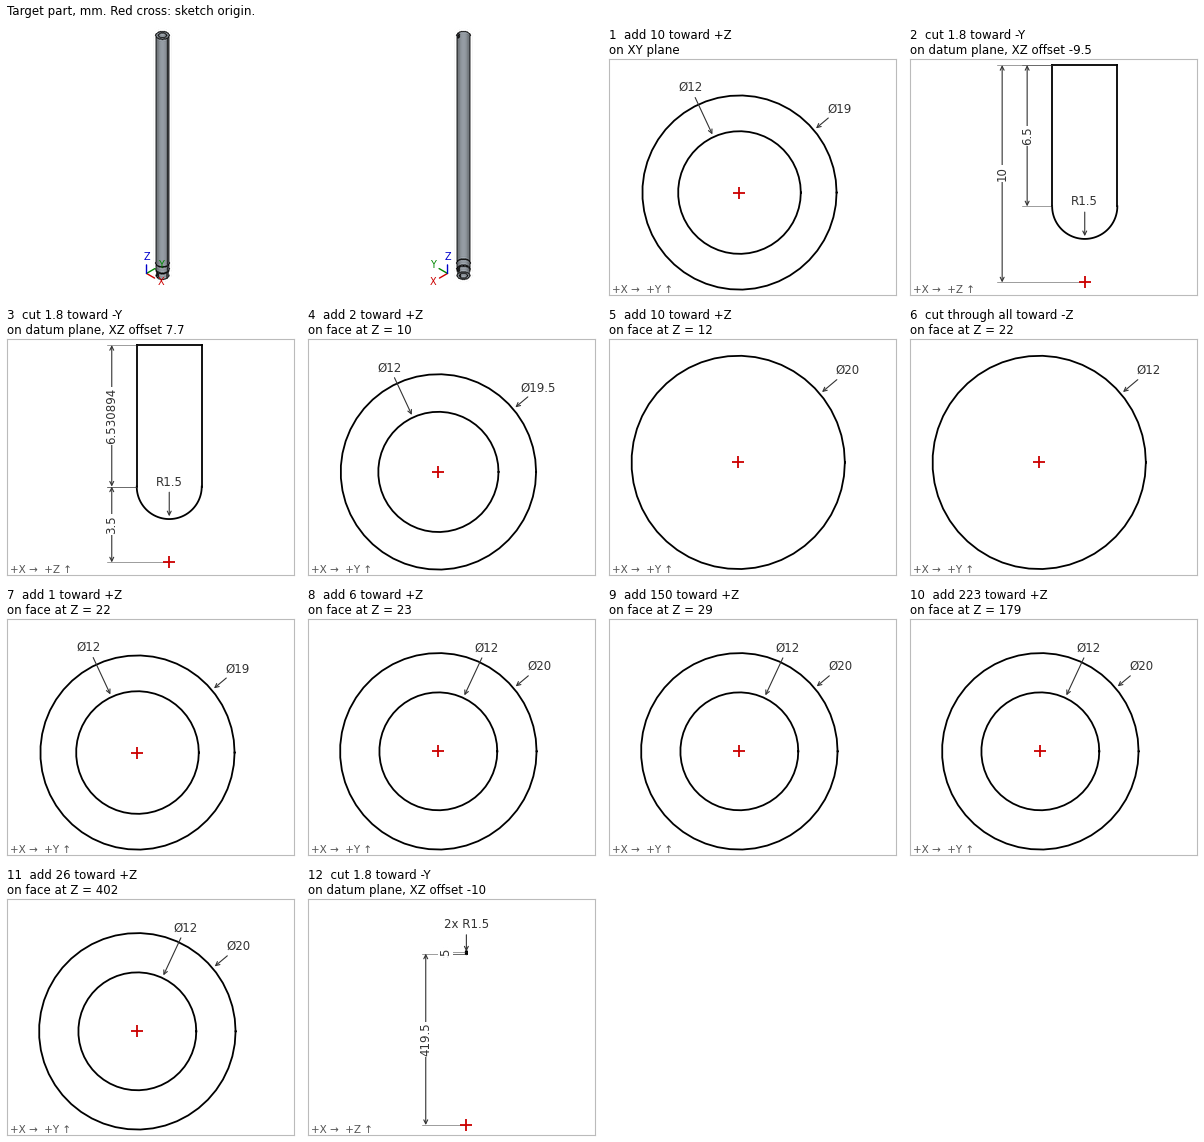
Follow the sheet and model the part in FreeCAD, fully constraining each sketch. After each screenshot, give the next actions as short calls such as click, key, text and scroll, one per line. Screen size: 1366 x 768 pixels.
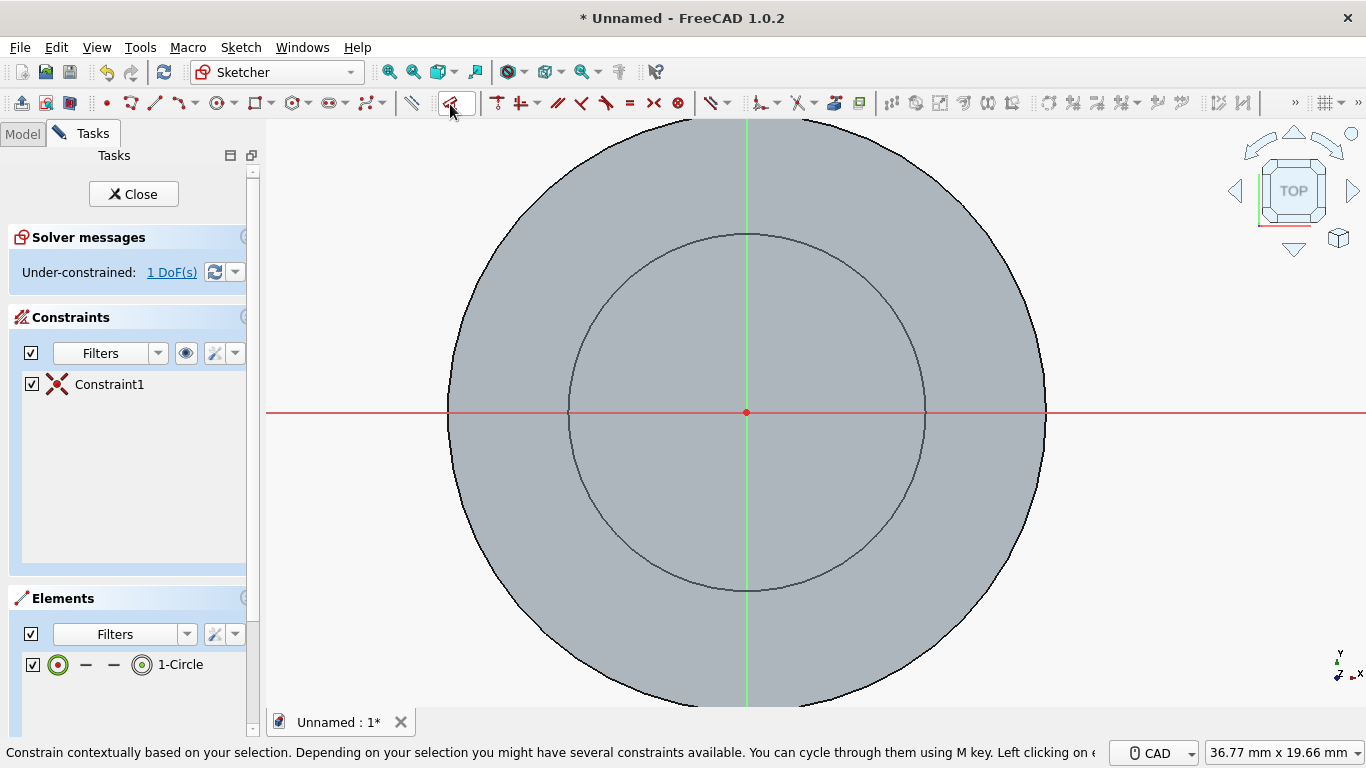
click(873, 286)
click(896, 263)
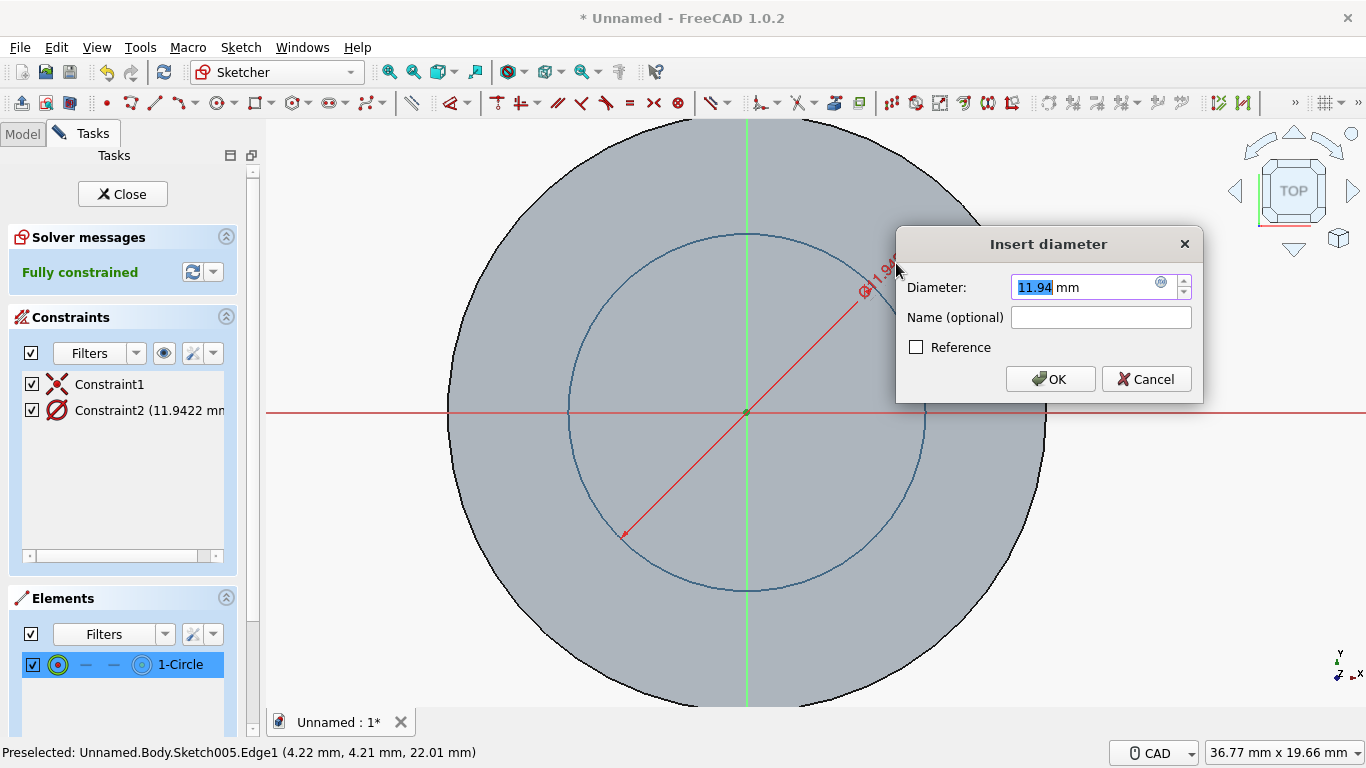
text(12)
key(Return)
key(Escape)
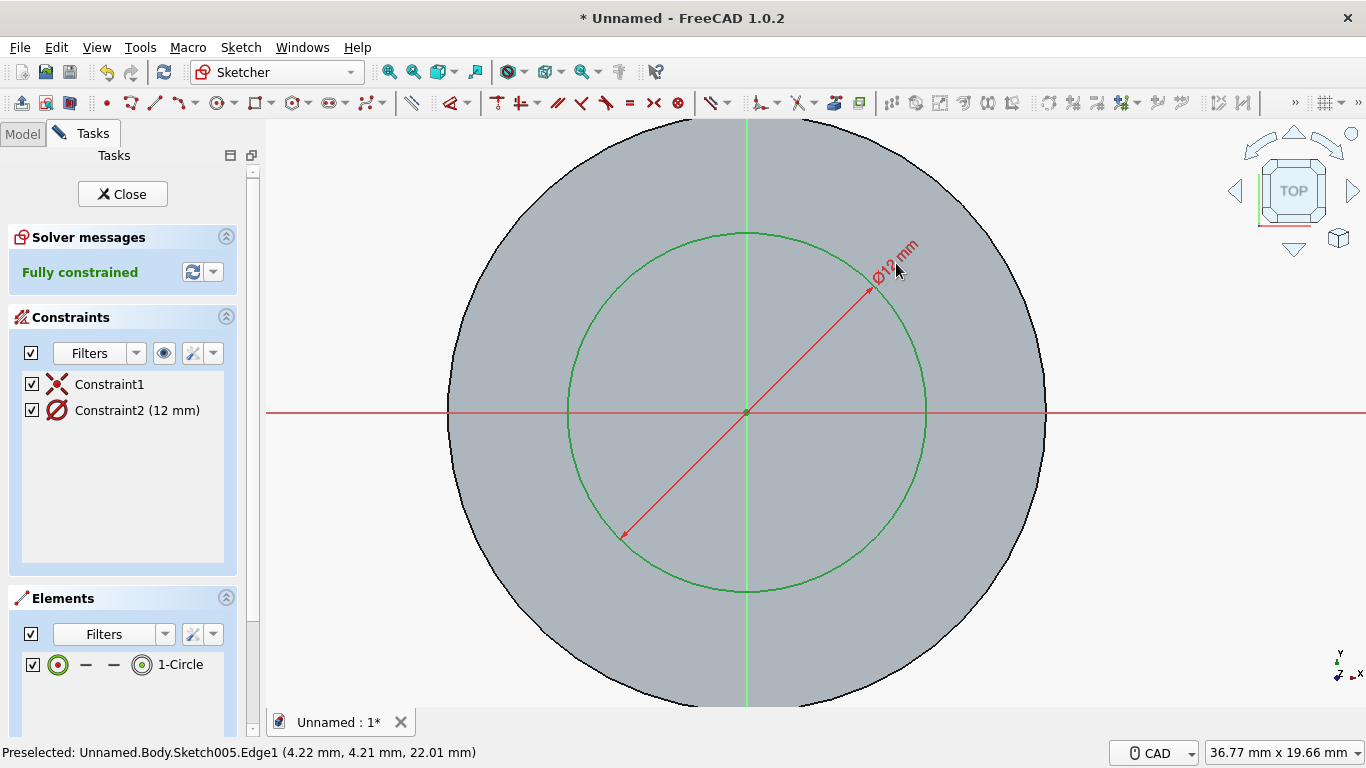
click(123, 194)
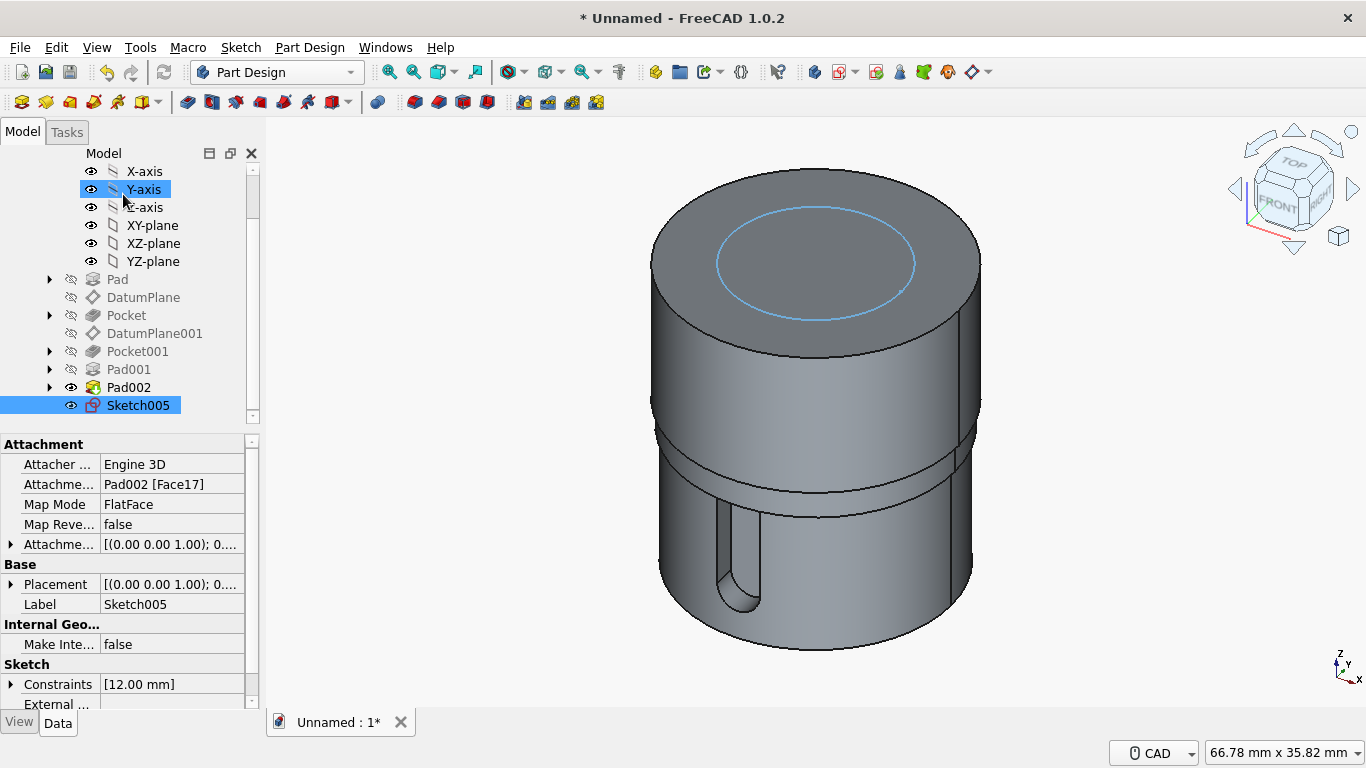
click(188, 102)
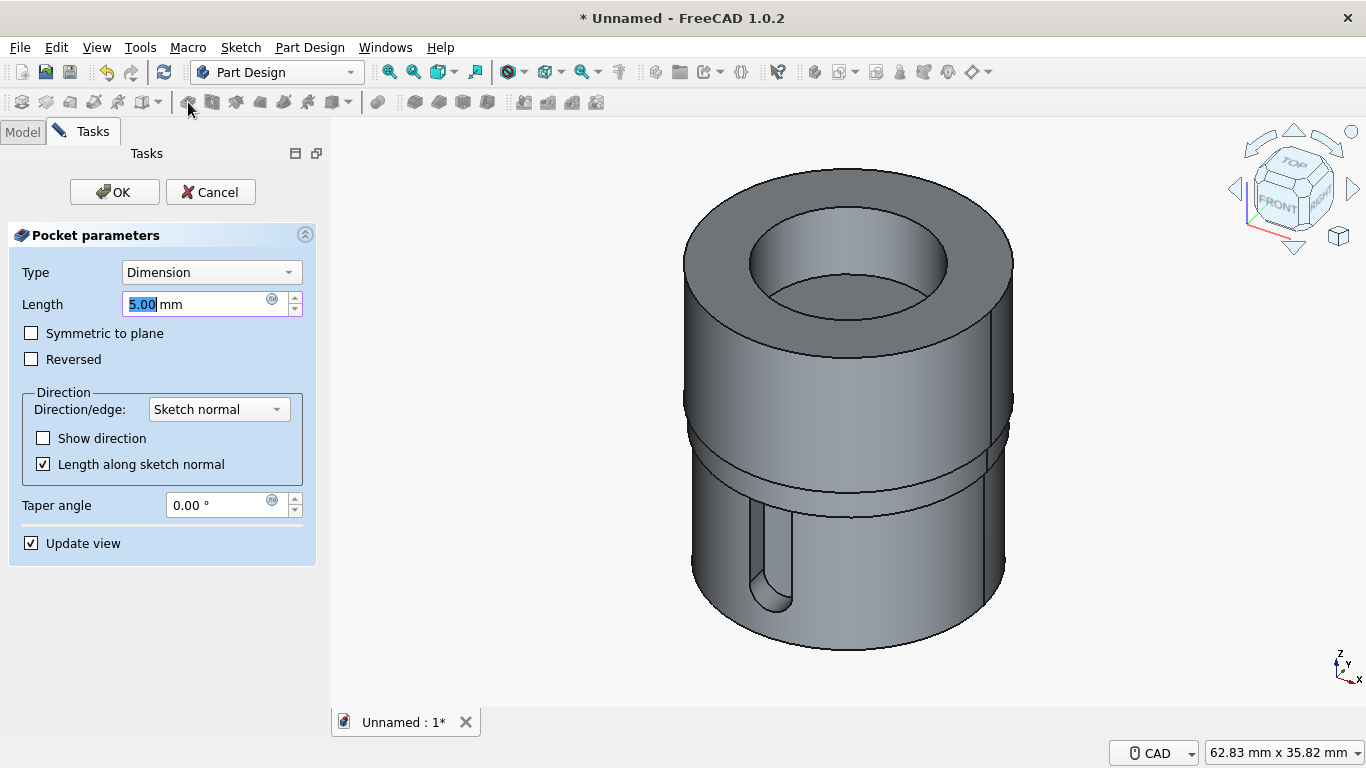
click(212, 272)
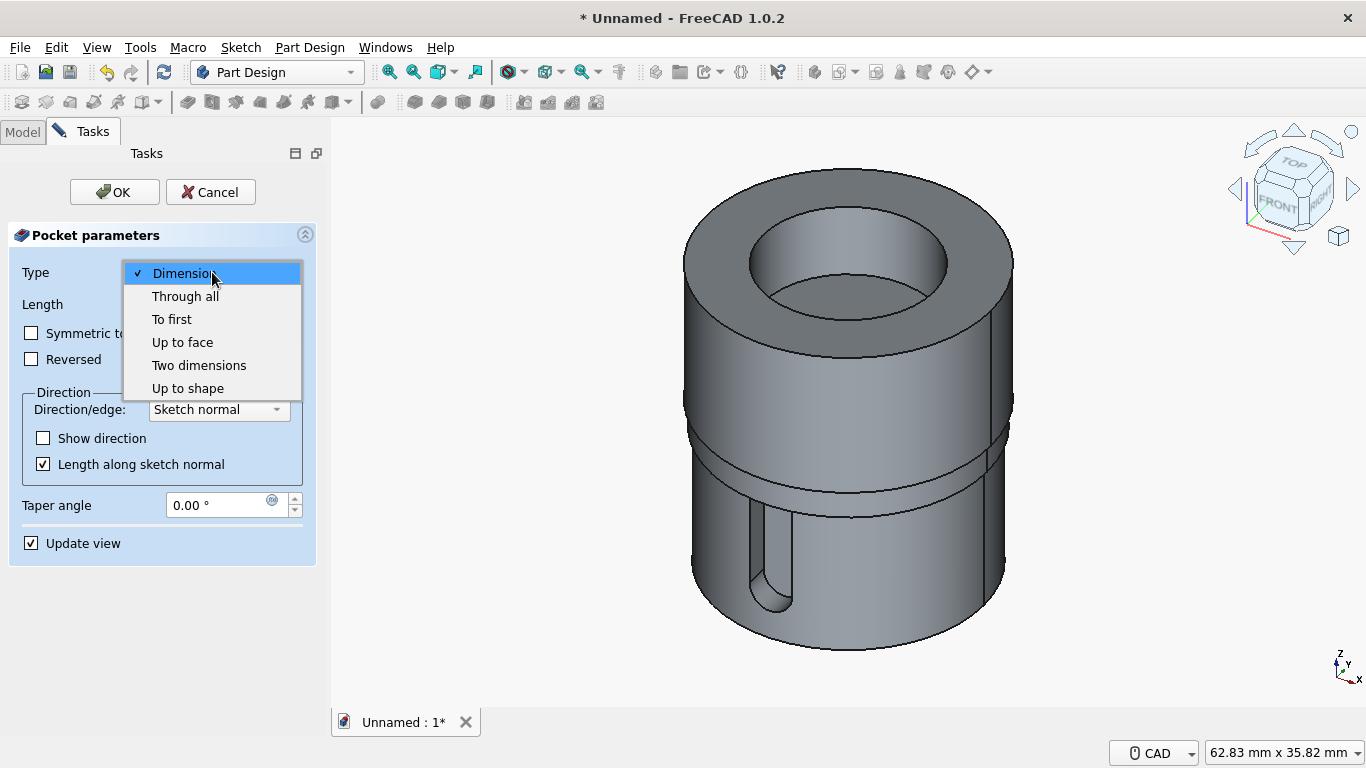
click(212, 296)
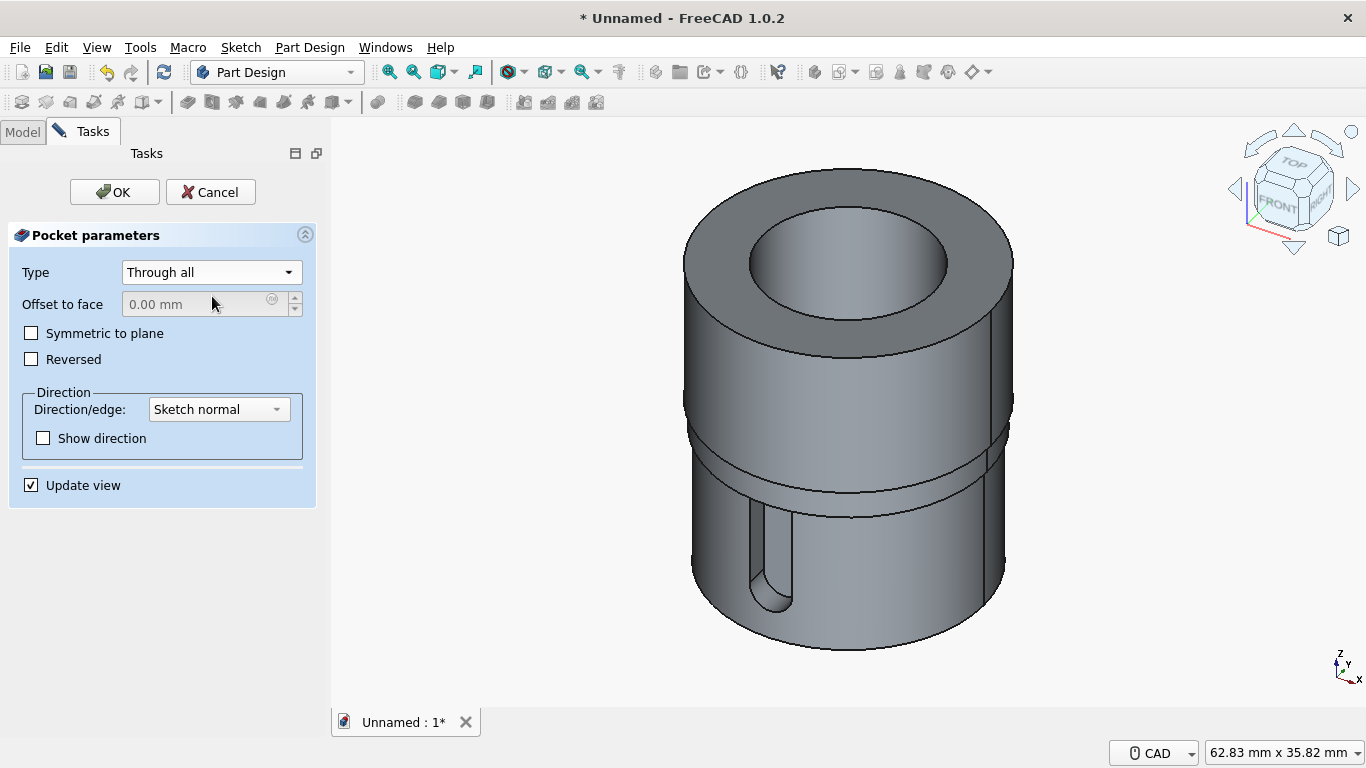
click(115, 192)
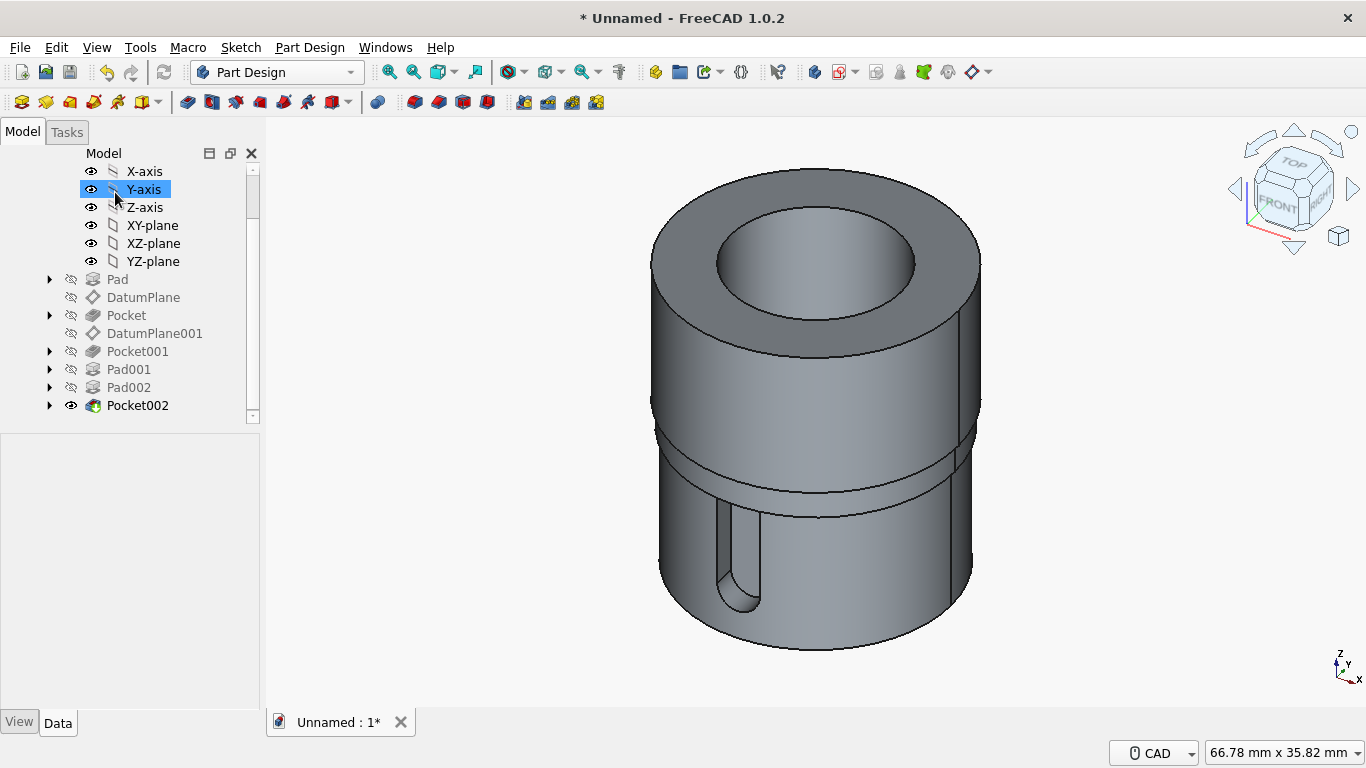
click(850, 336)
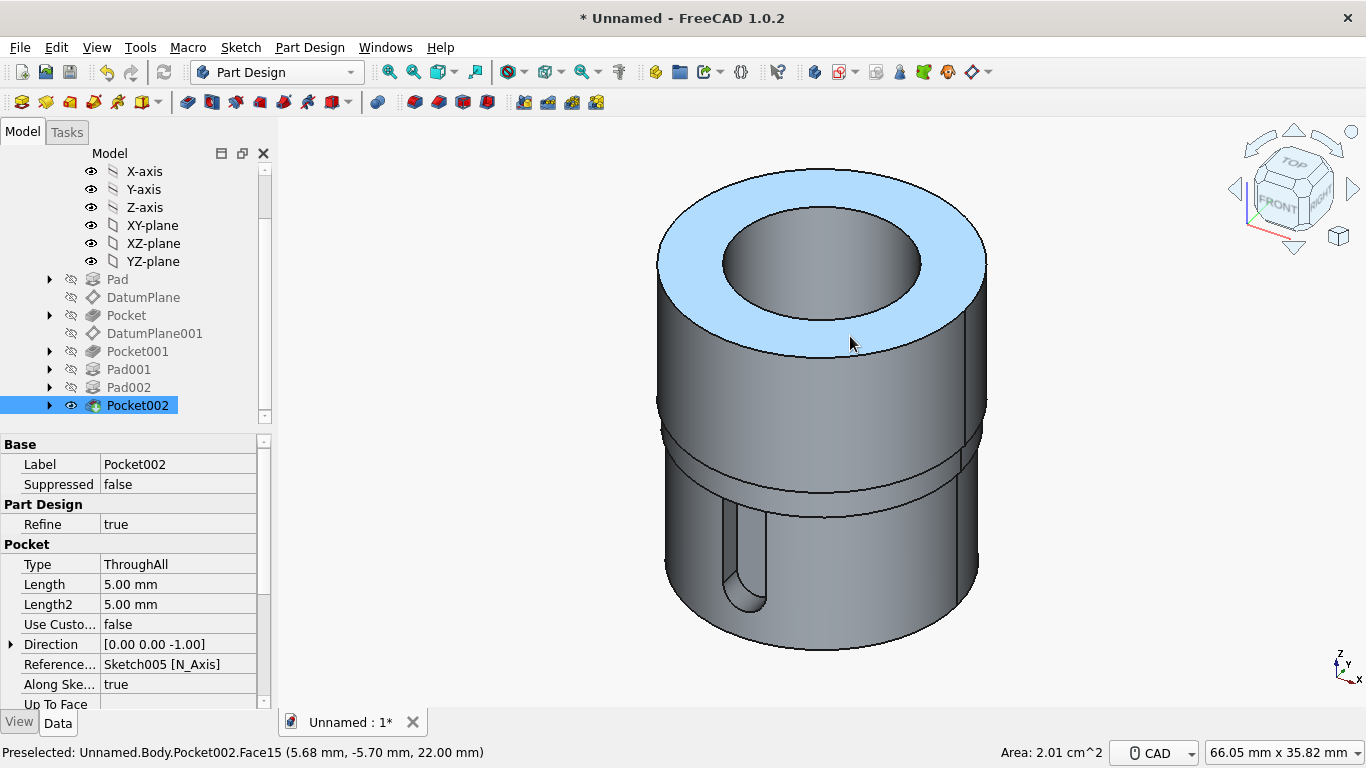
click(840, 72)